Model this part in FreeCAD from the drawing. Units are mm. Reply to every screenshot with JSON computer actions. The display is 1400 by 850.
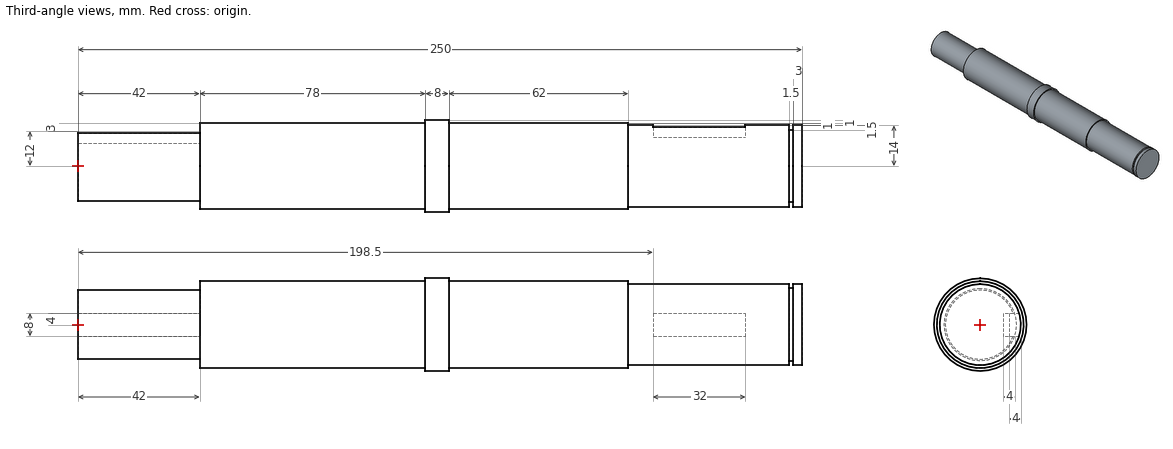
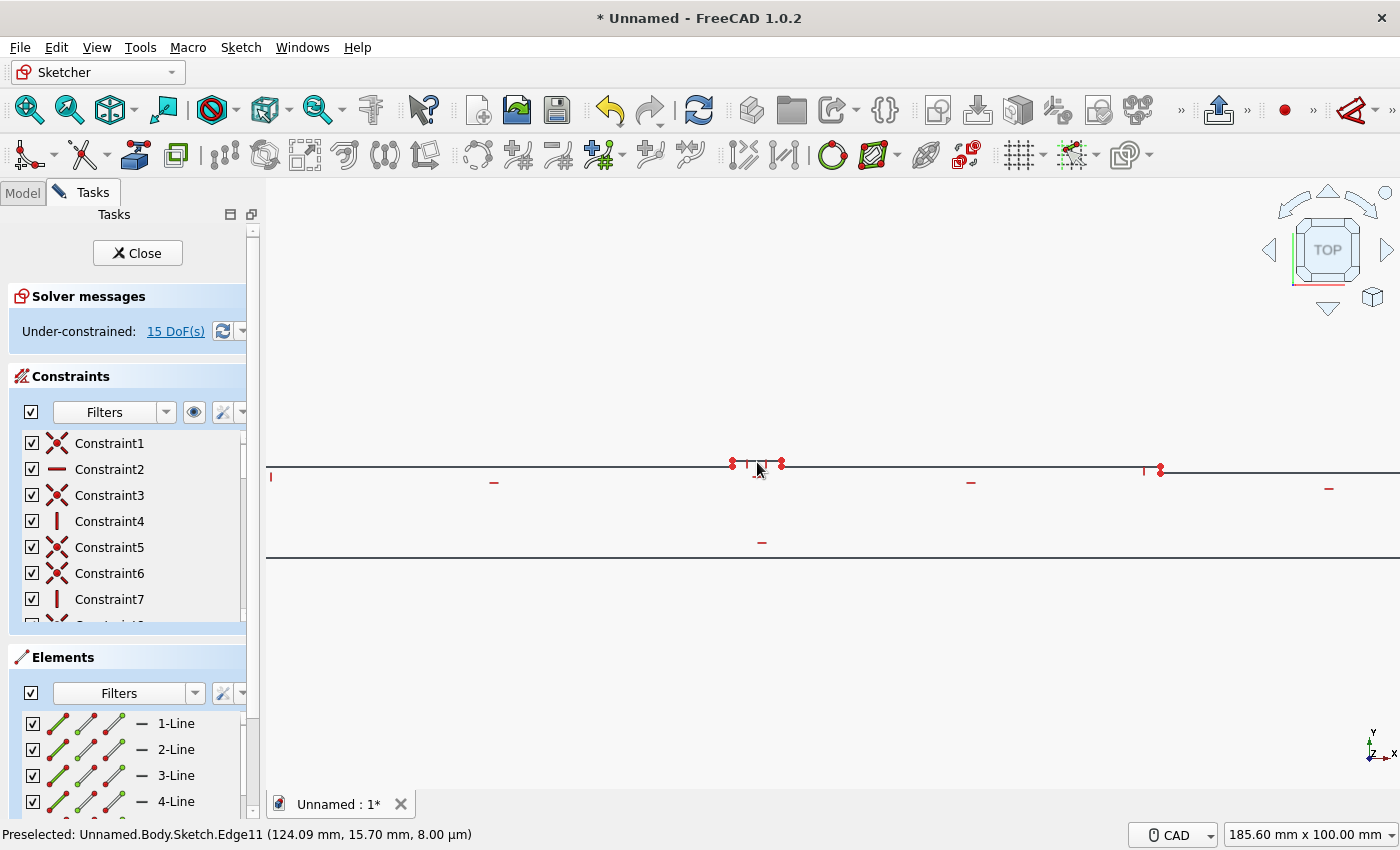
{"action": "scroll", "coordinate": [766, 462], "scroll_direction": "down", "scroll_amount": 4}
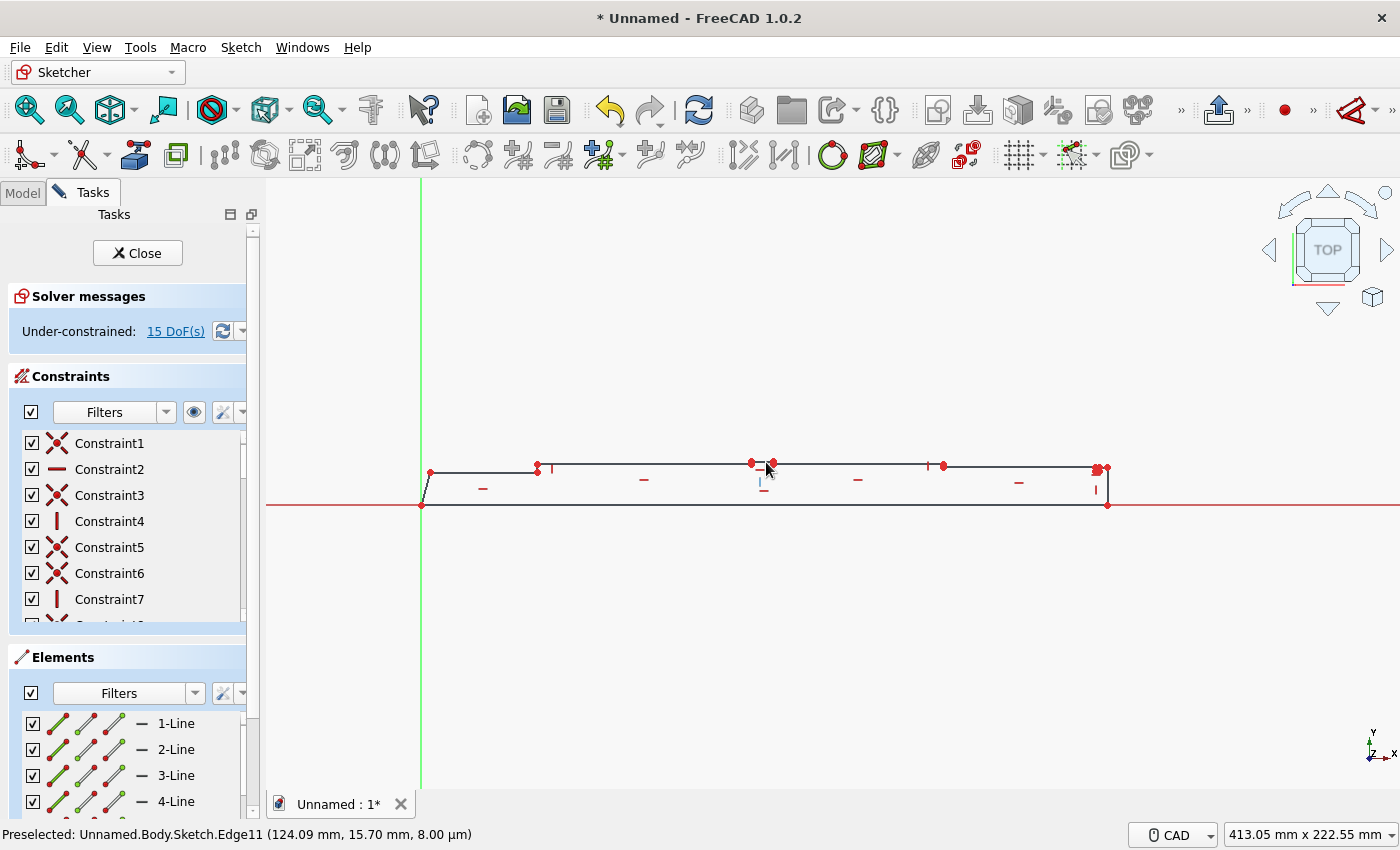
{"action": "scroll", "coordinate": [428, 483], "scroll_direction": "up", "scroll_amount": 5}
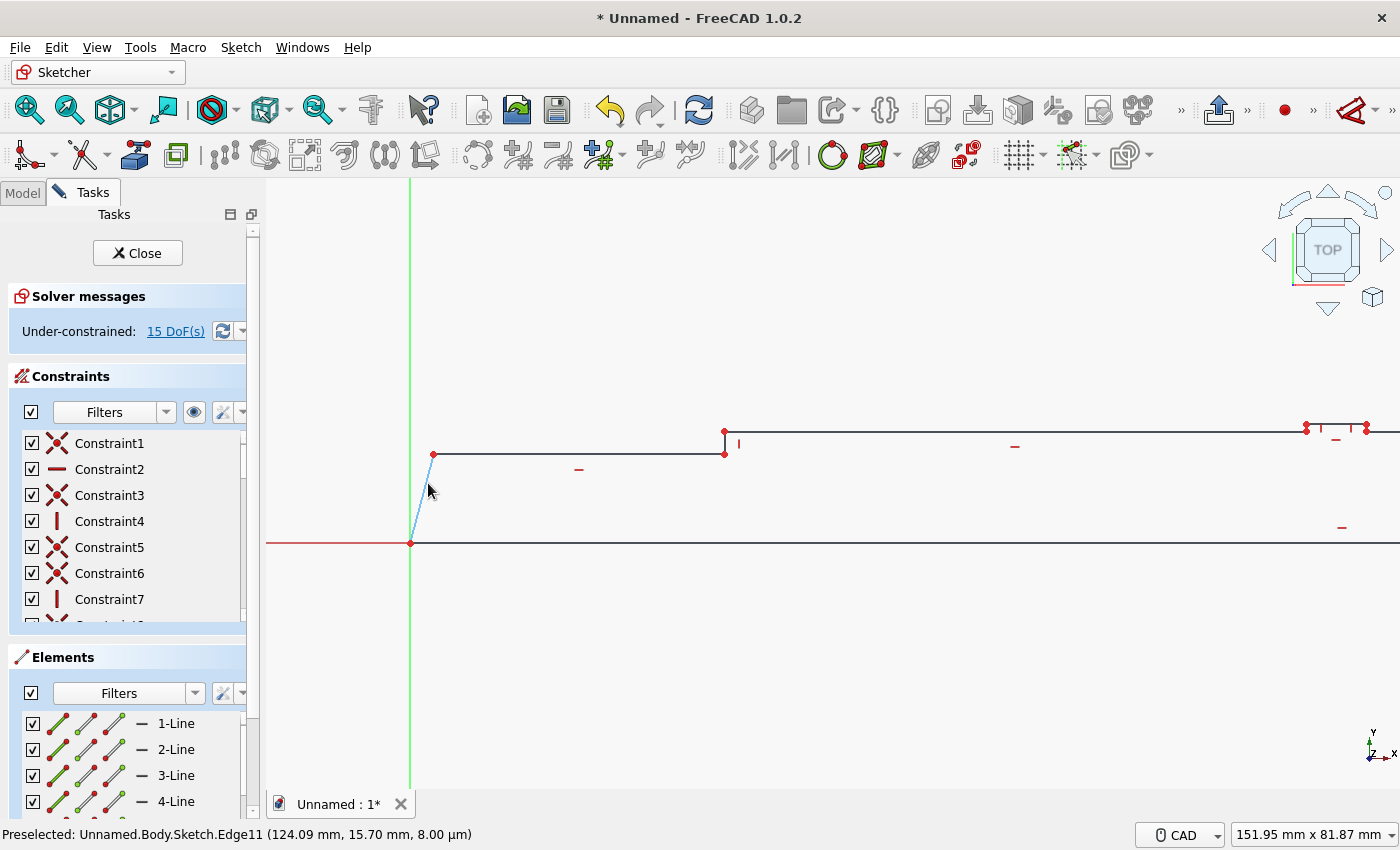
{"action": "left_click", "coordinate": [427, 481]}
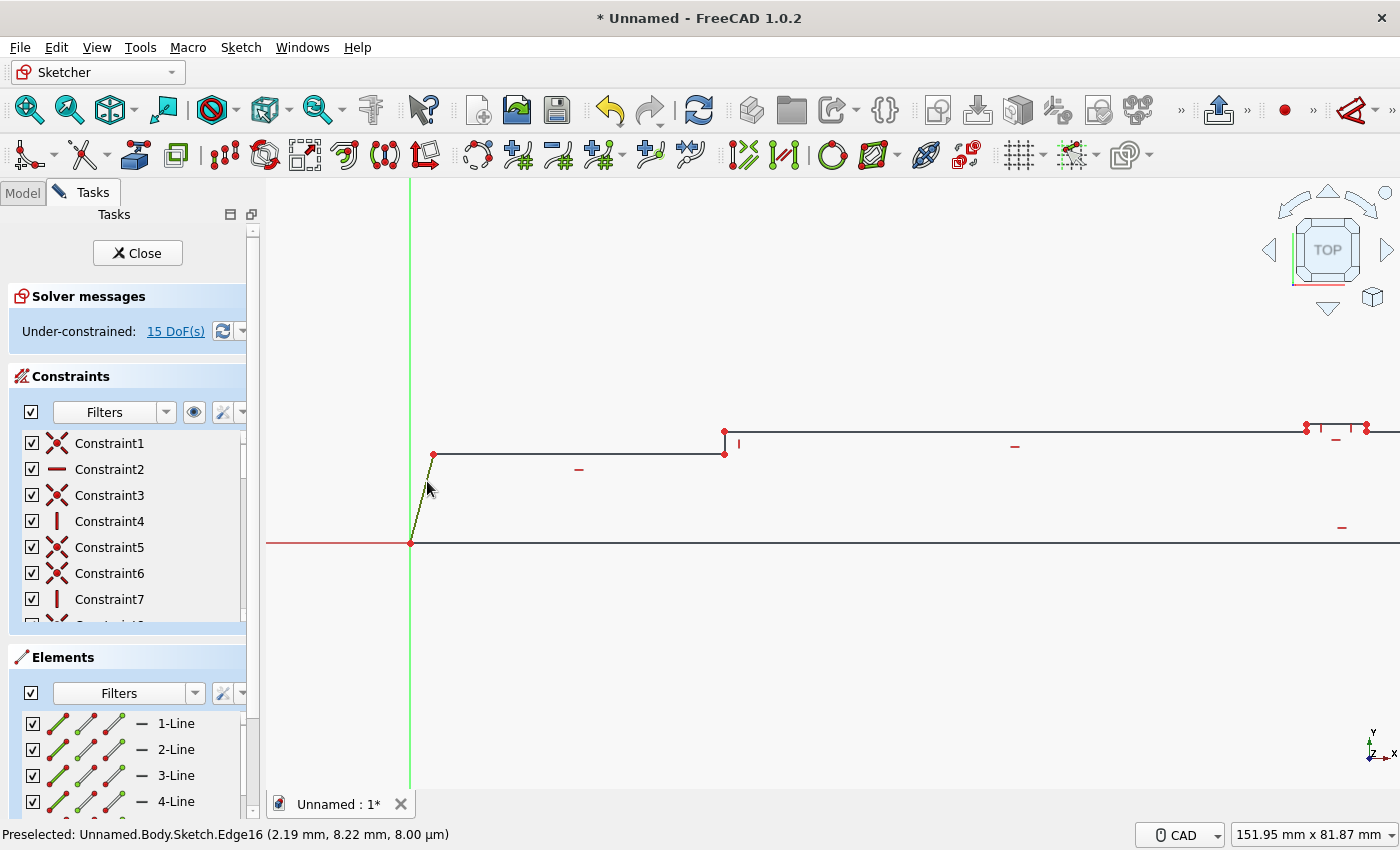
{"action": "key", "text": "v"}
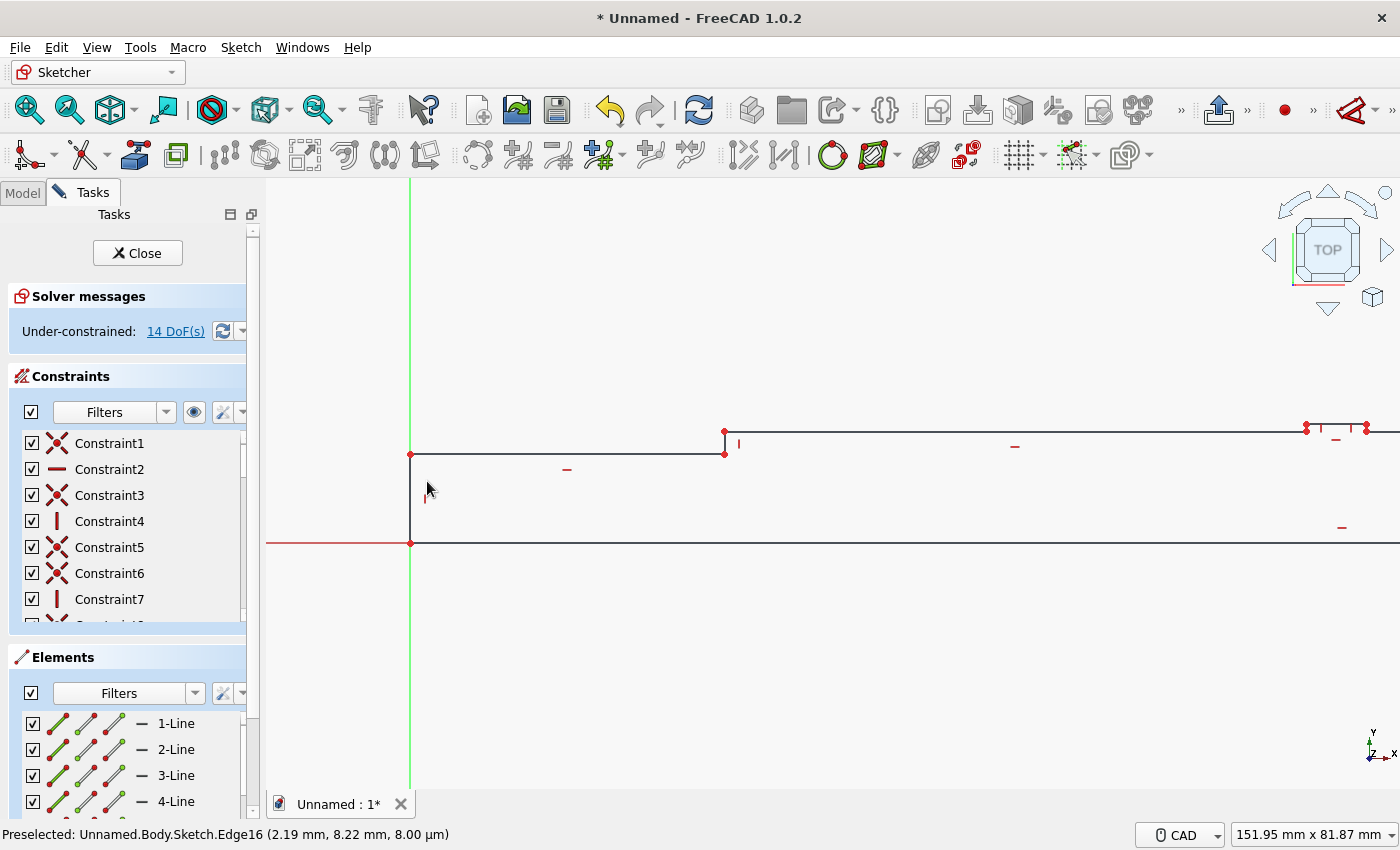
{"action": "scroll", "coordinate": [428, 483], "scroll_direction": "down", "scroll_amount": 5}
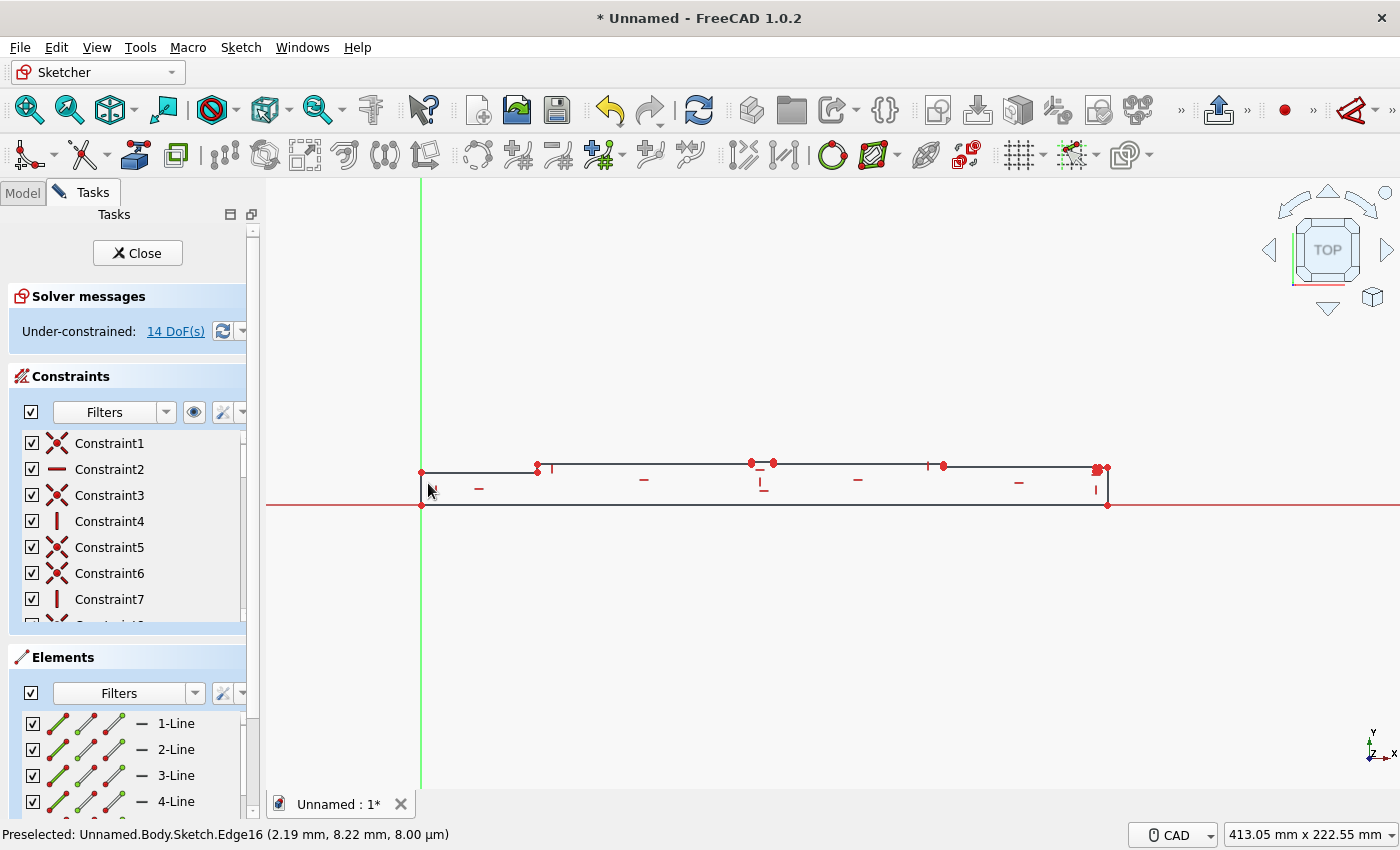
{"action": "scroll", "coordinate": [1104, 468], "scroll_direction": "up", "scroll_amount": 8}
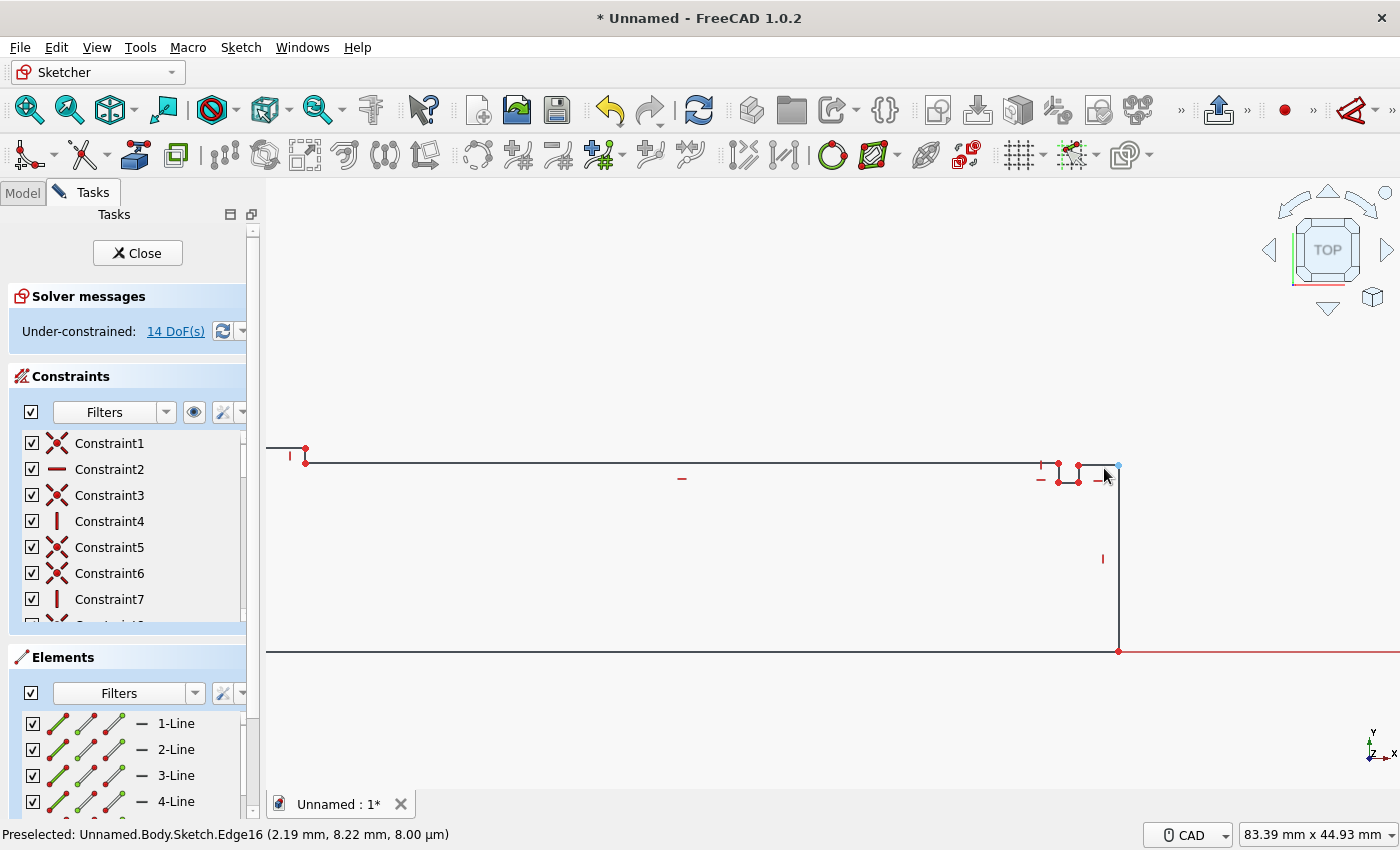
{"action": "left_click", "coordinate": [1099, 465]}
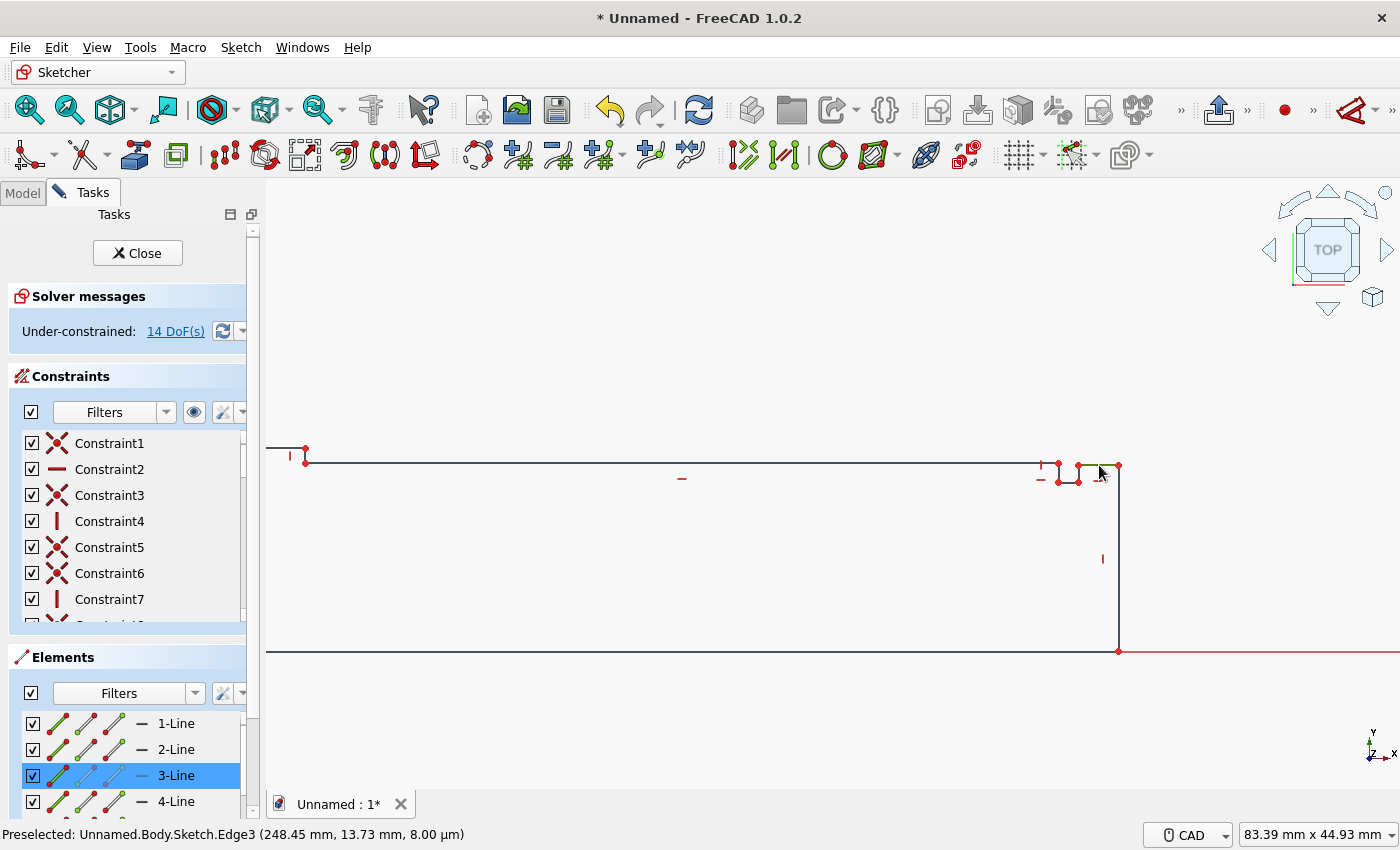
{"action": "key", "text": "l"}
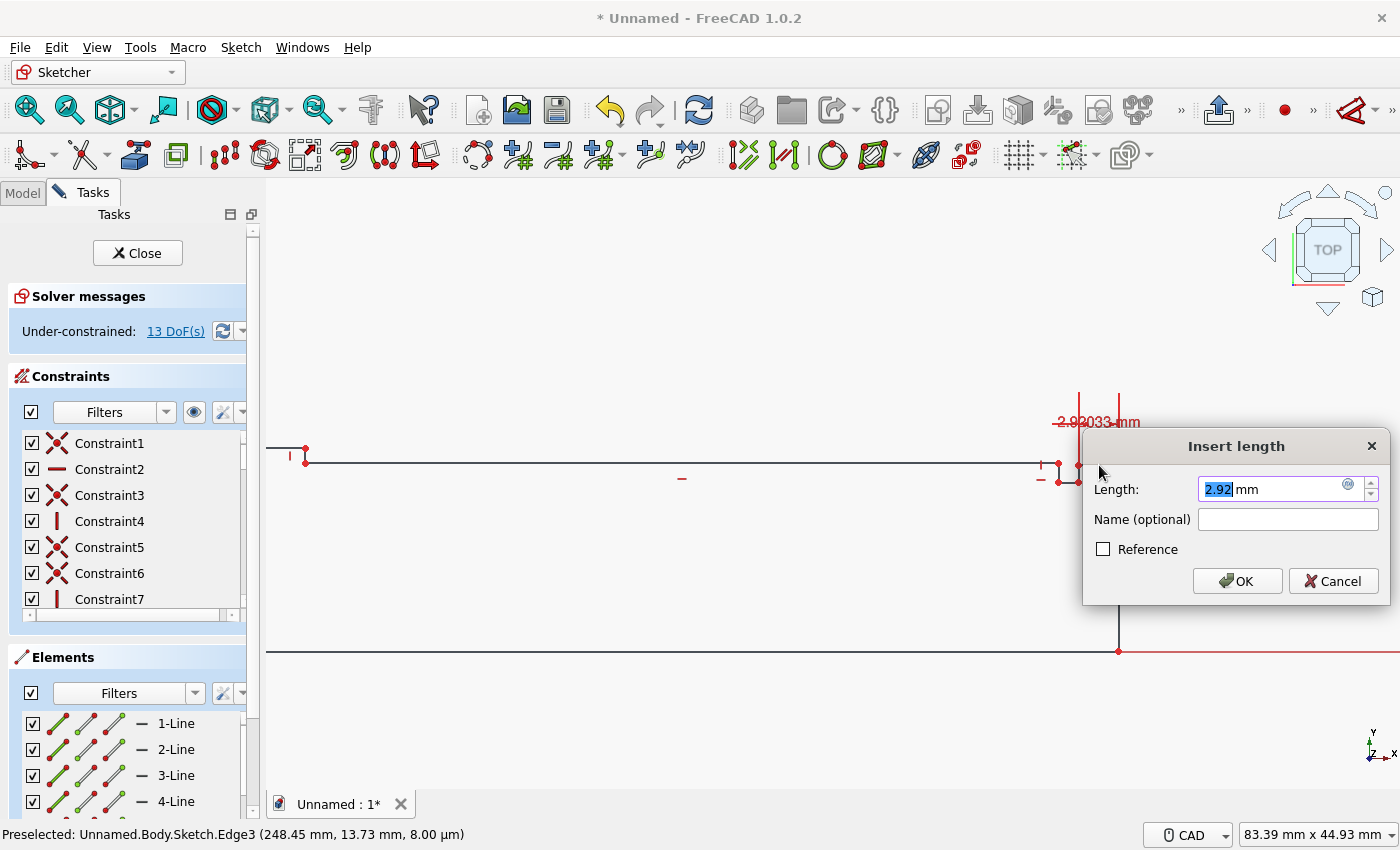
{"action": "type", "text": "3"}
{"action": "key", "text": "Return"}